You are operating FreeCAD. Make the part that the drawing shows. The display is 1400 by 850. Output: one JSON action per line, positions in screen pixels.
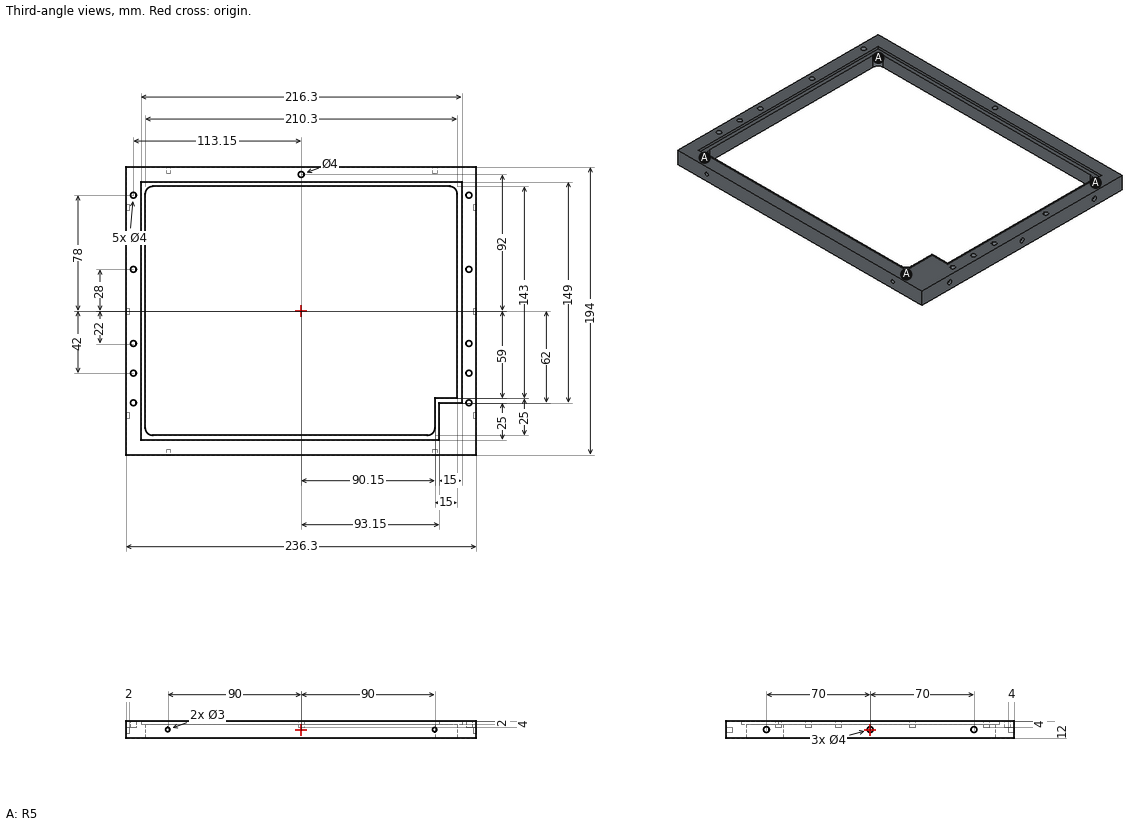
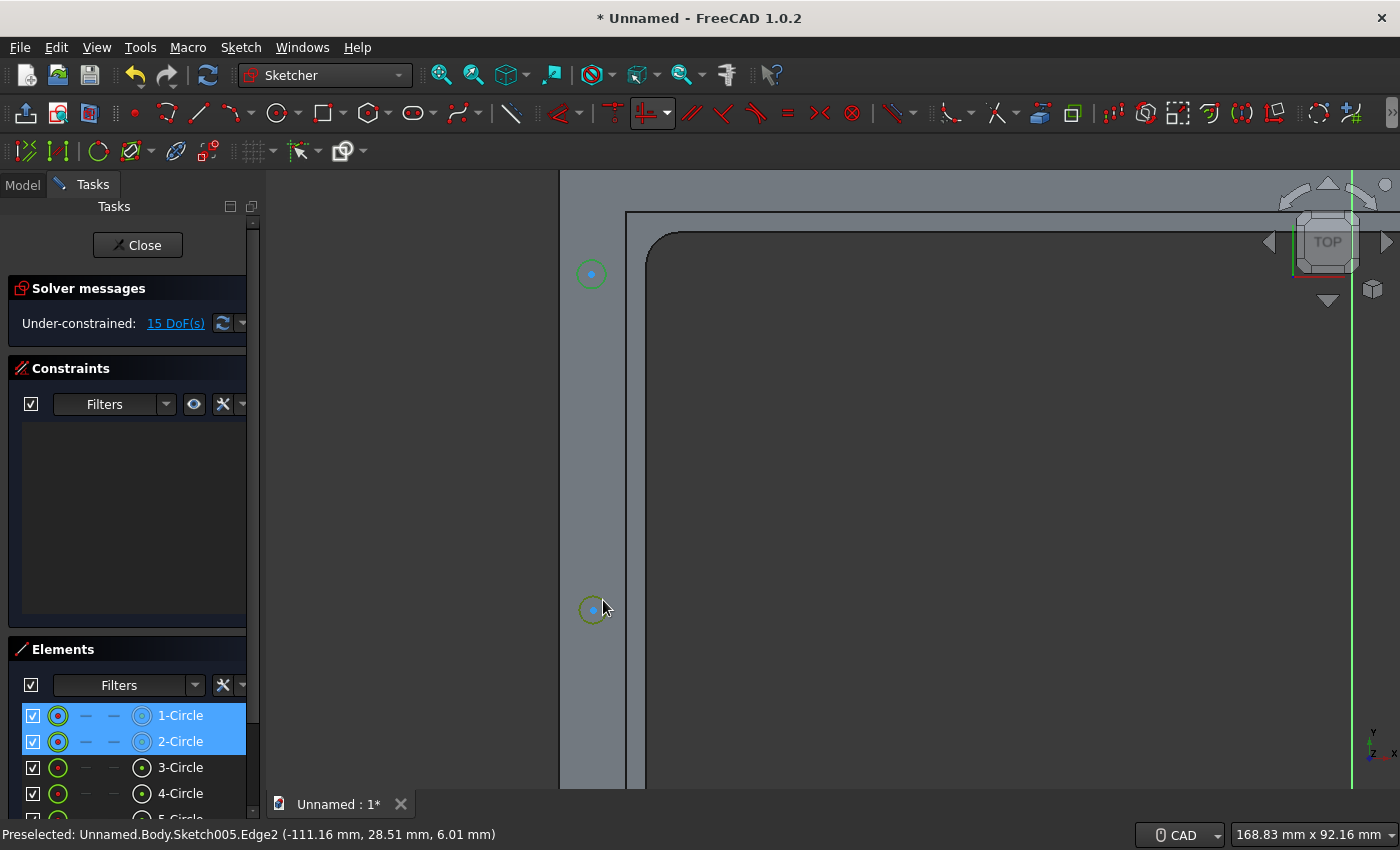
{"action": "scroll", "coordinate": [600, 265], "scroll_direction": "down", "scroll_amount": 4}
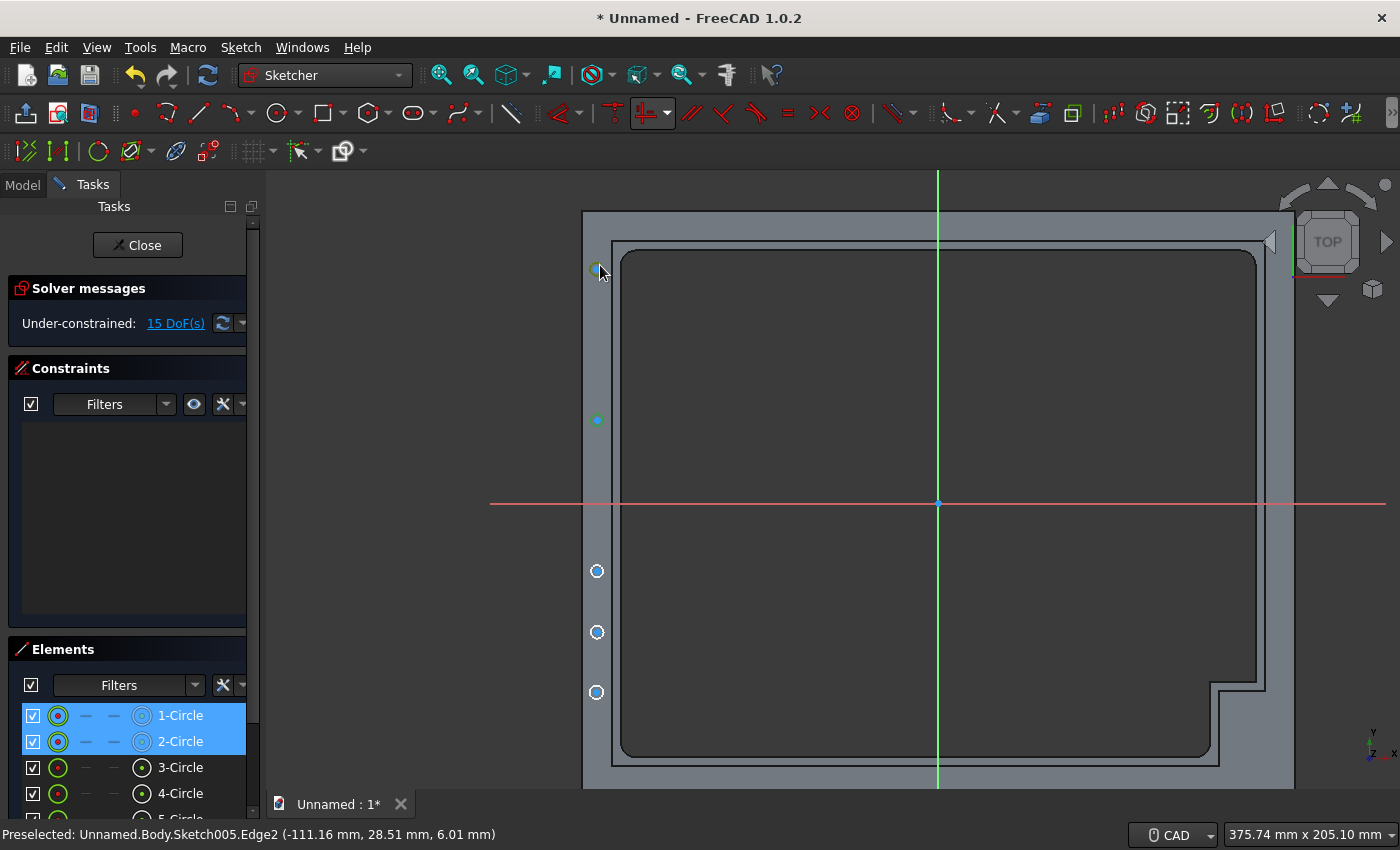
{"action": "scroll", "coordinate": [601, 567], "scroll_direction": "up", "scroll_amount": 5}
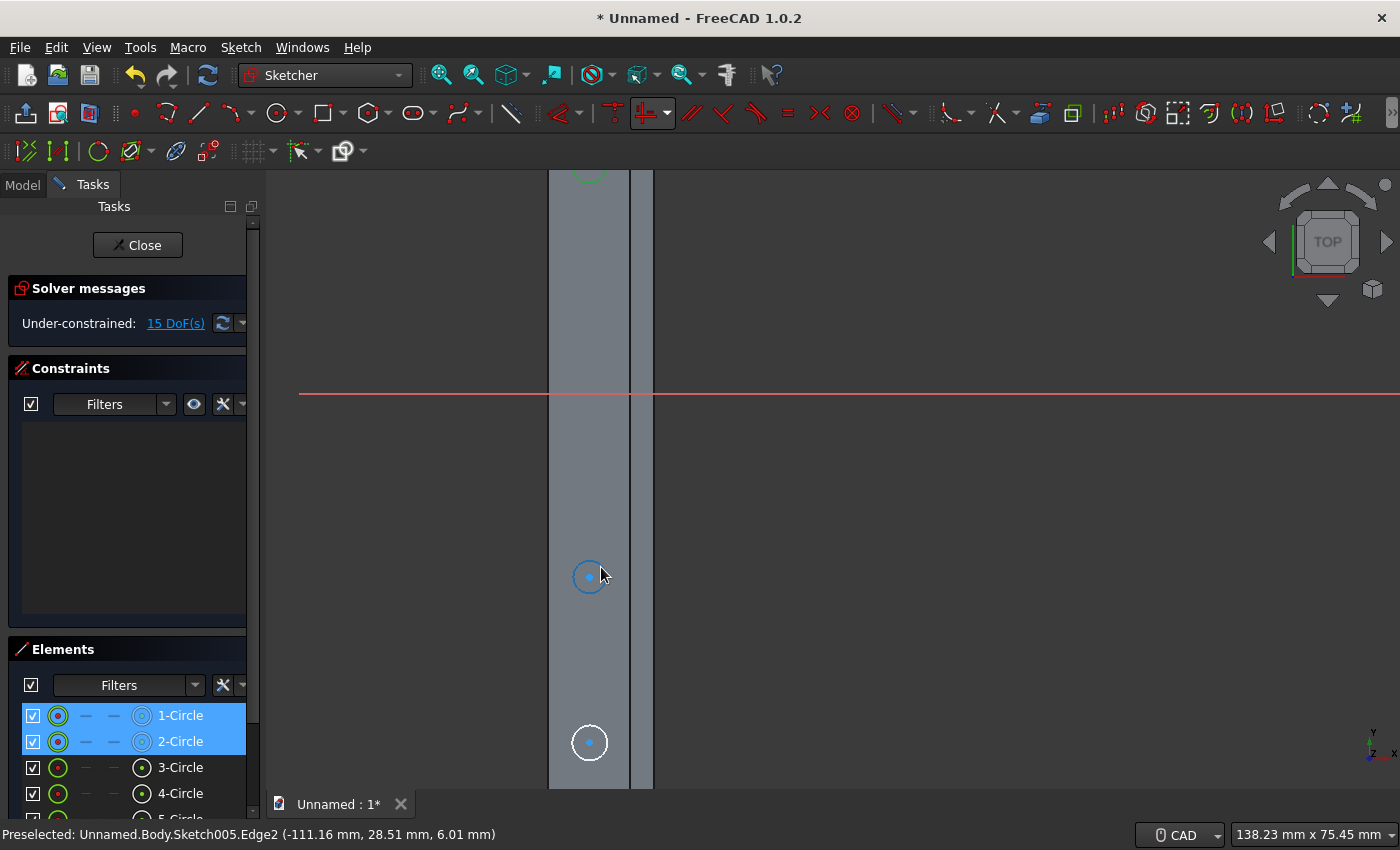
{"action": "left_click", "coordinate": [601, 566]}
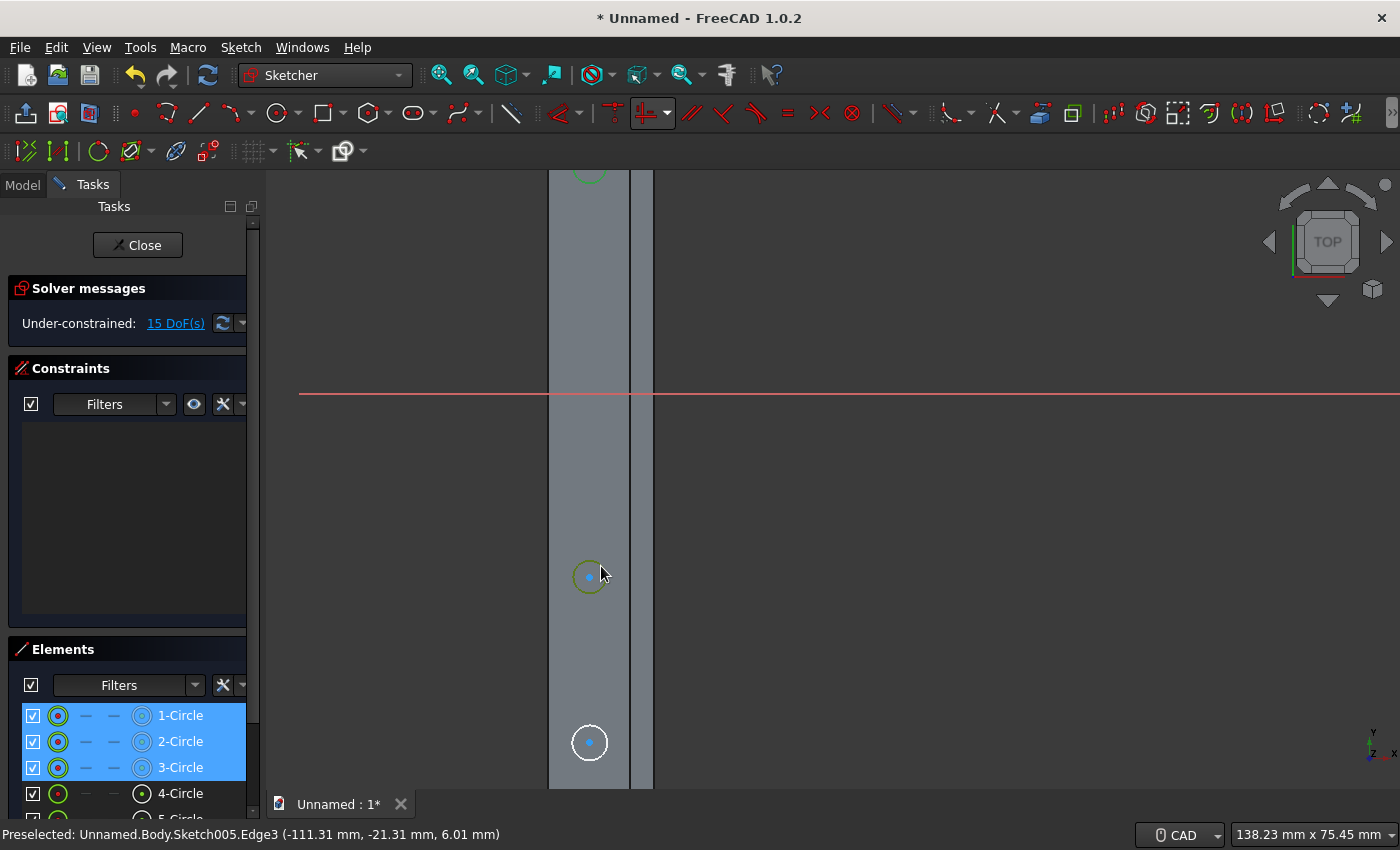
{"action": "left_click", "coordinate": [602, 731]}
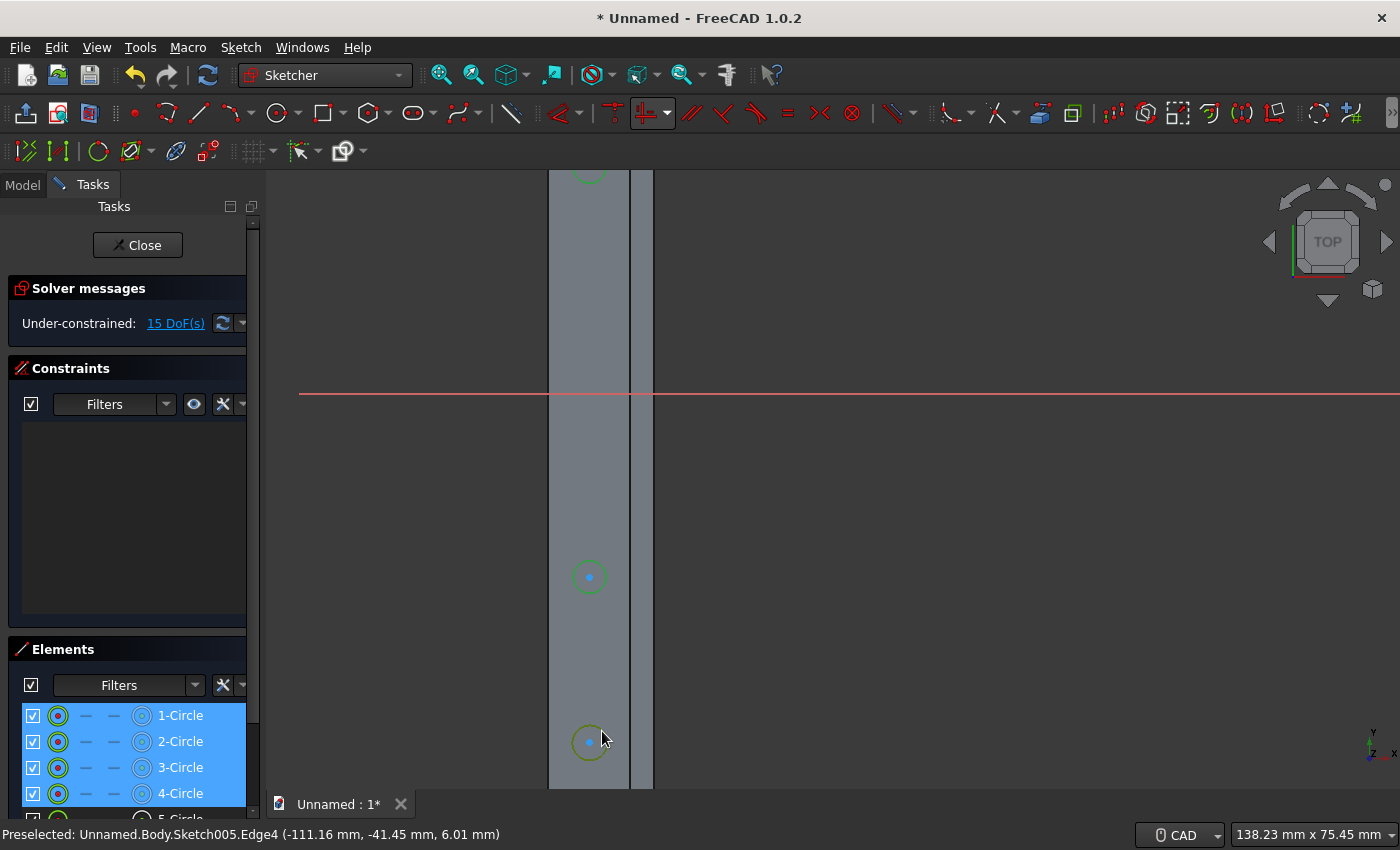
{"action": "scroll", "coordinate": [601, 567], "scroll_direction": "down", "scroll_amount": 5}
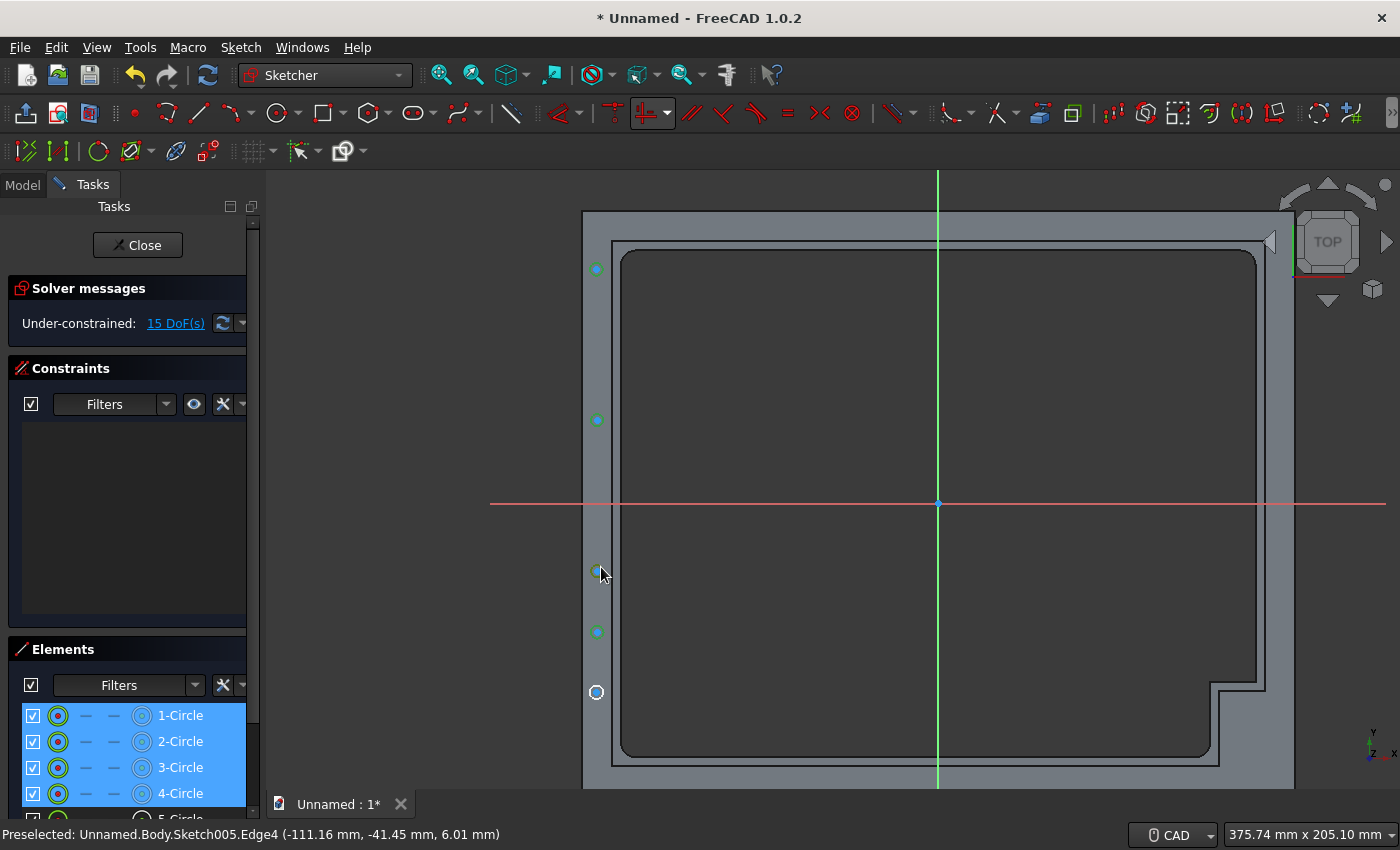
{"action": "scroll", "coordinate": [601, 688], "scroll_direction": "up", "scroll_amount": 4}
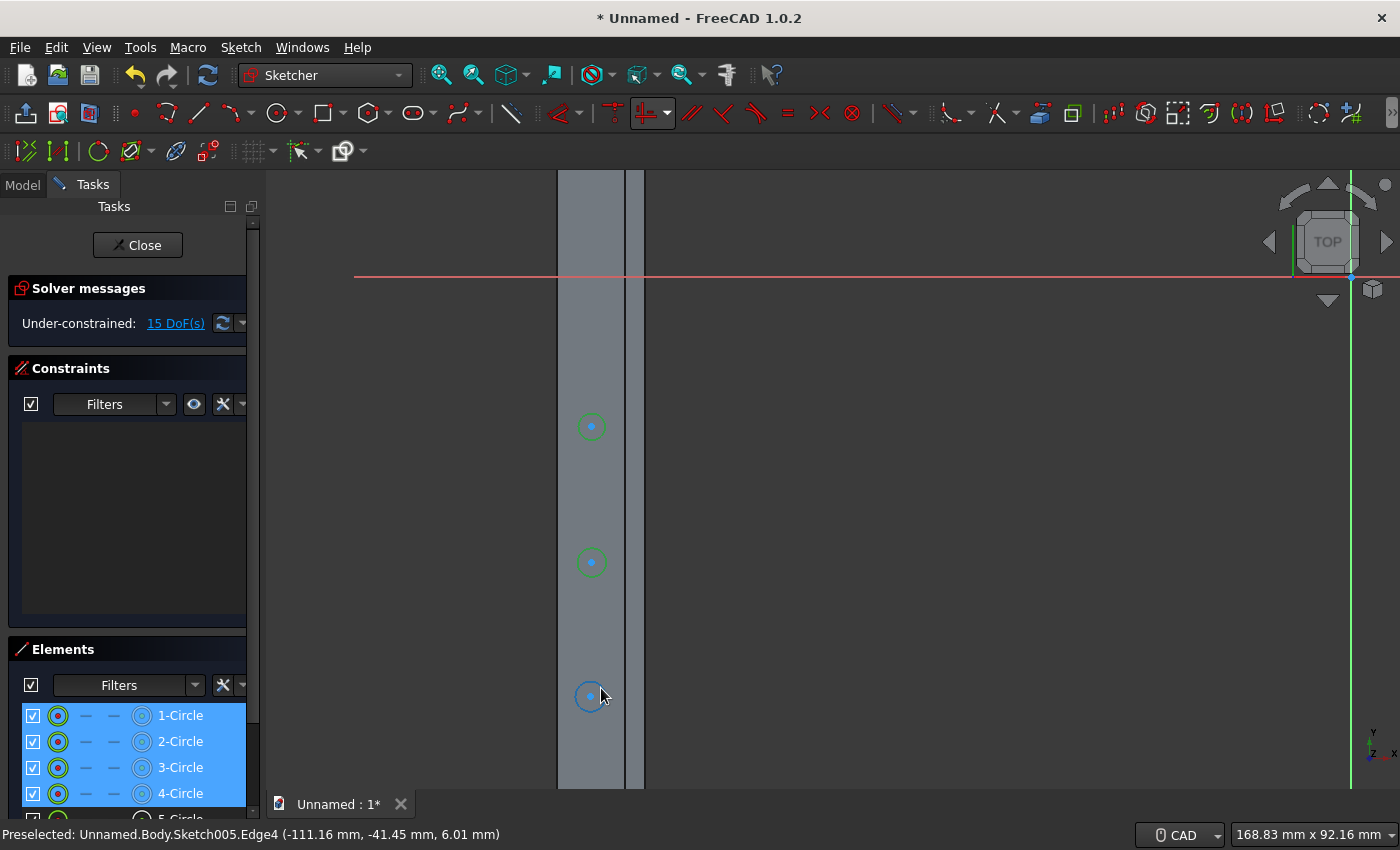
{"action": "left_click", "coordinate": [601, 686]}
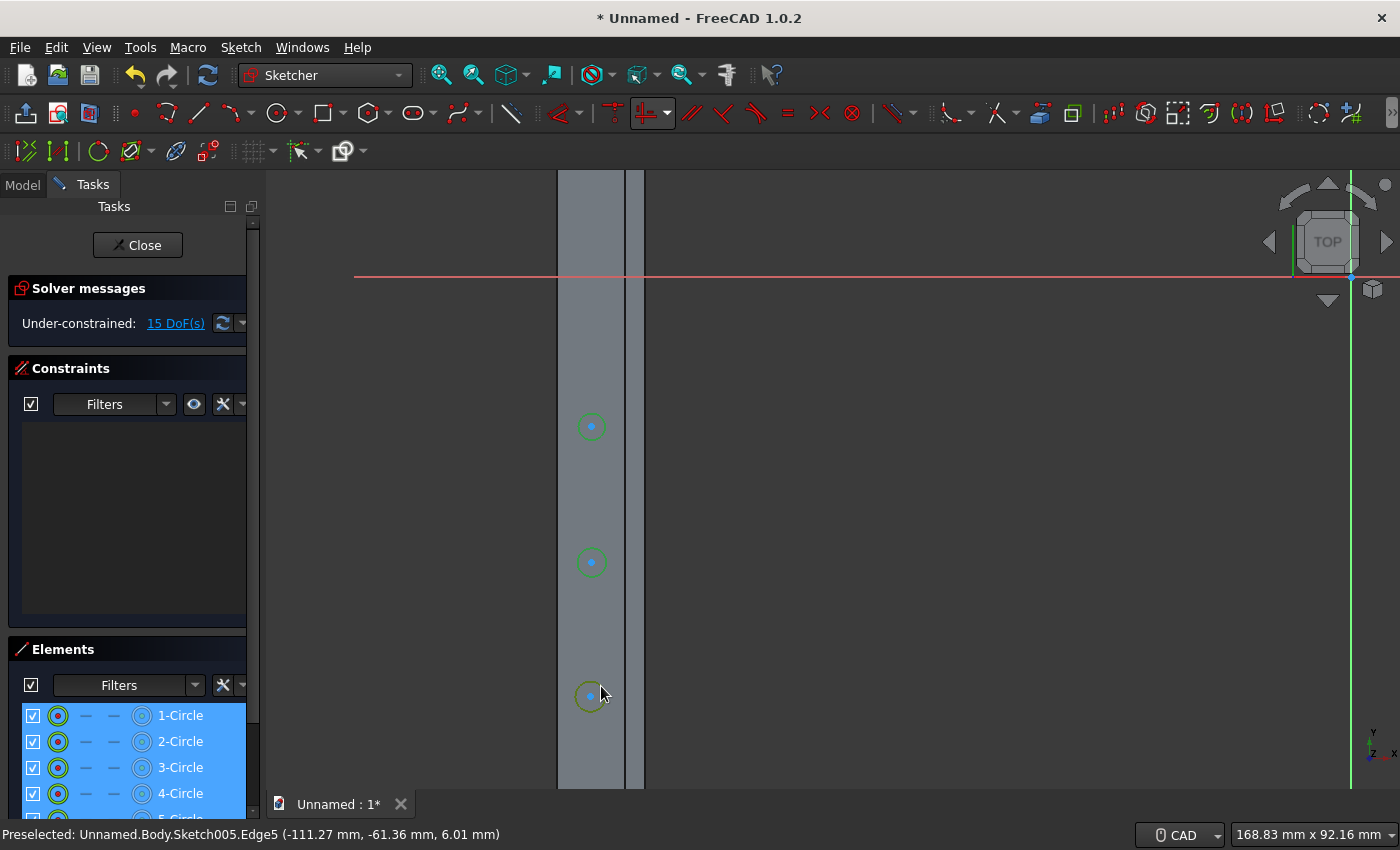
{"action": "left_click", "coordinate": [788, 114]}